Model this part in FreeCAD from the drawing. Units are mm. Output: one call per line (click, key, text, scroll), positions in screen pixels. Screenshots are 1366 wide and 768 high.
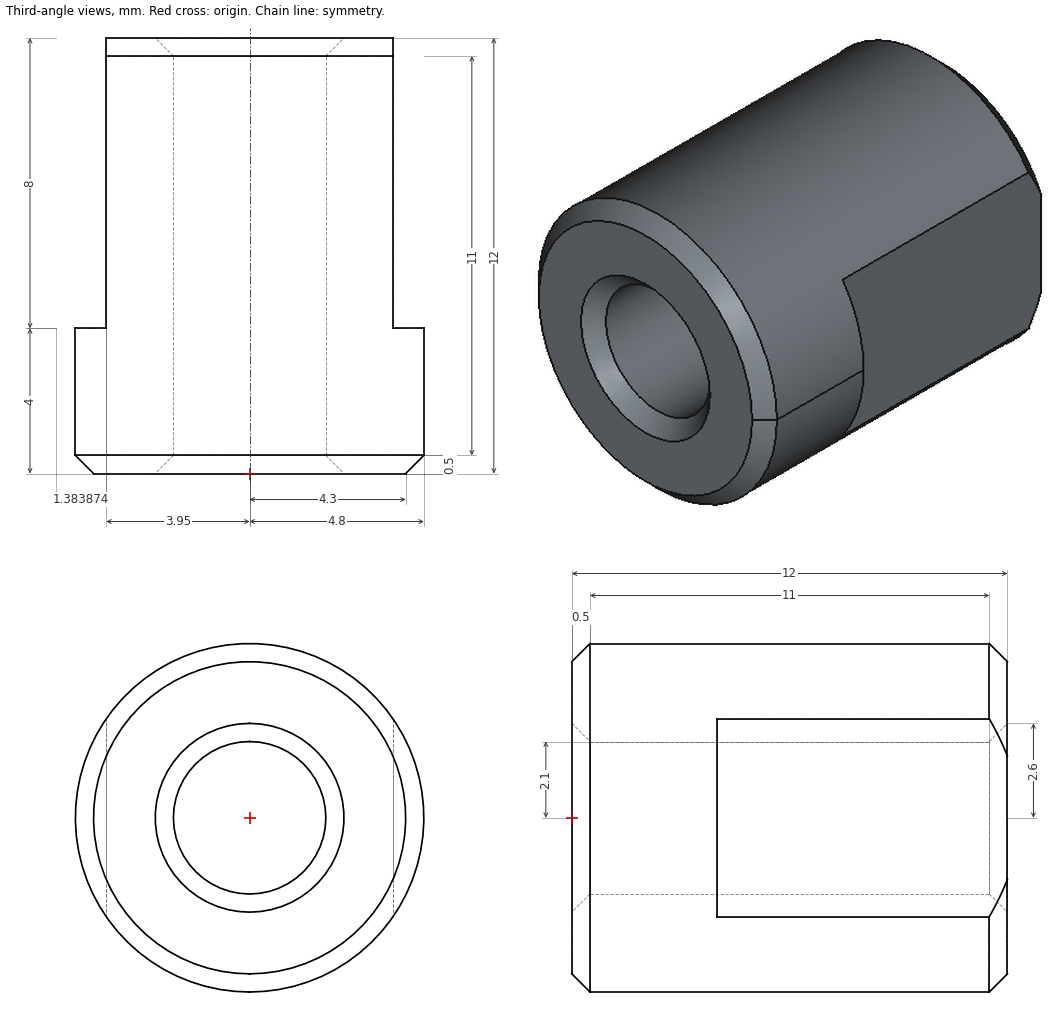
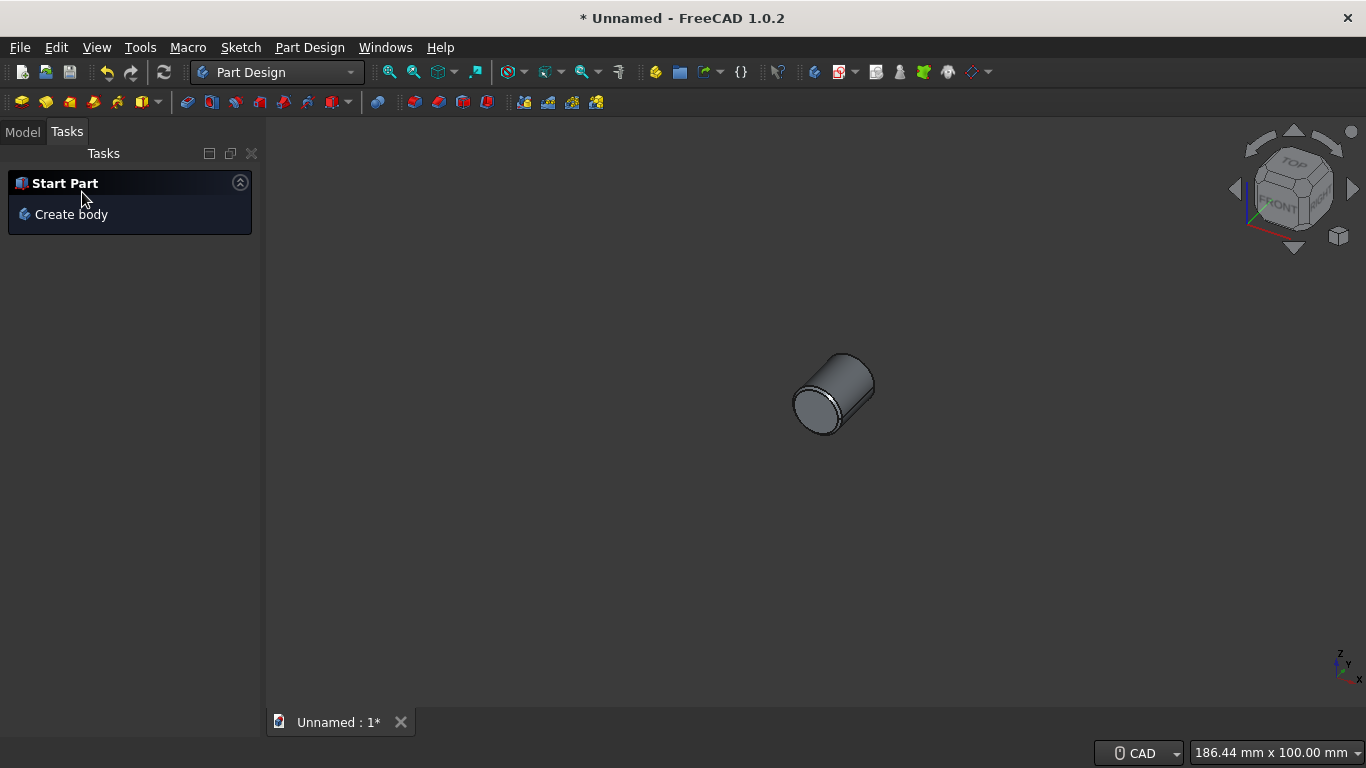
click(390, 72)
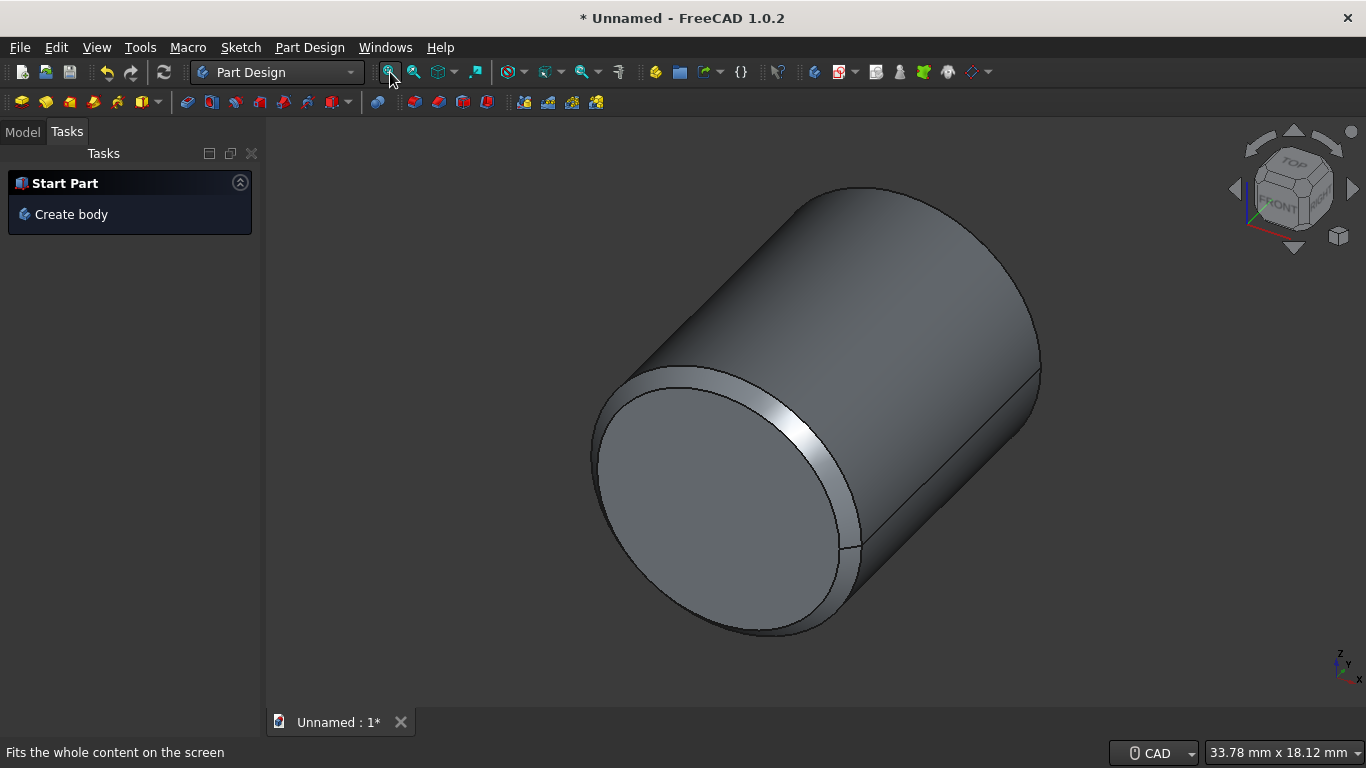
click(840, 72)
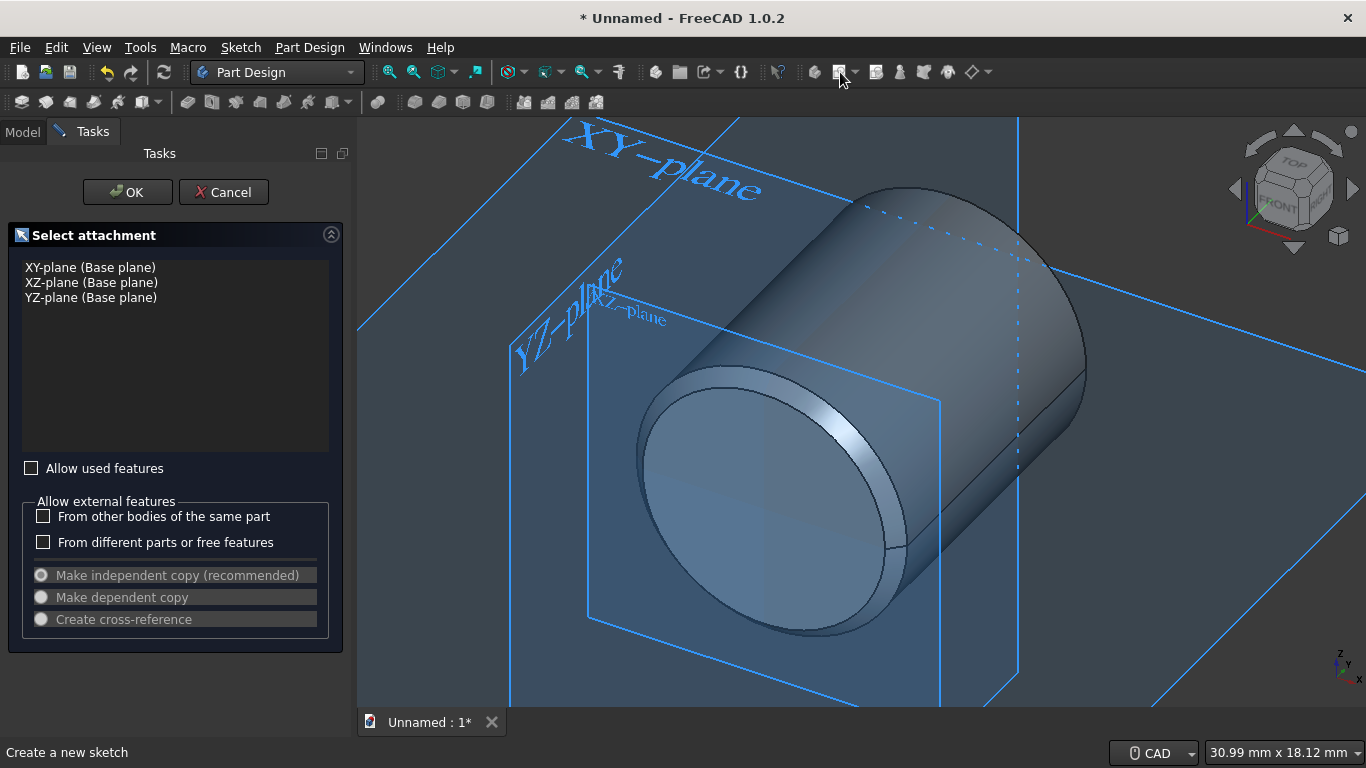
click(82, 298)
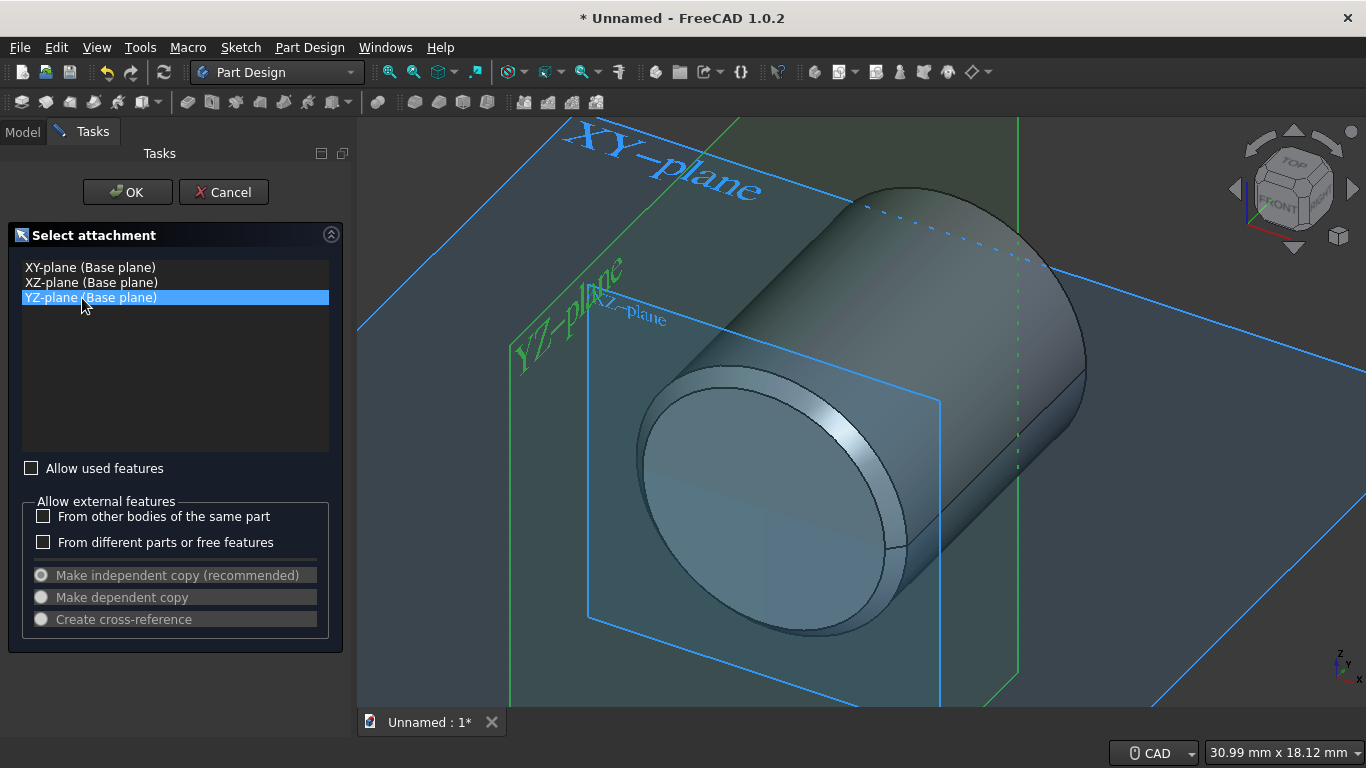
click(128, 192)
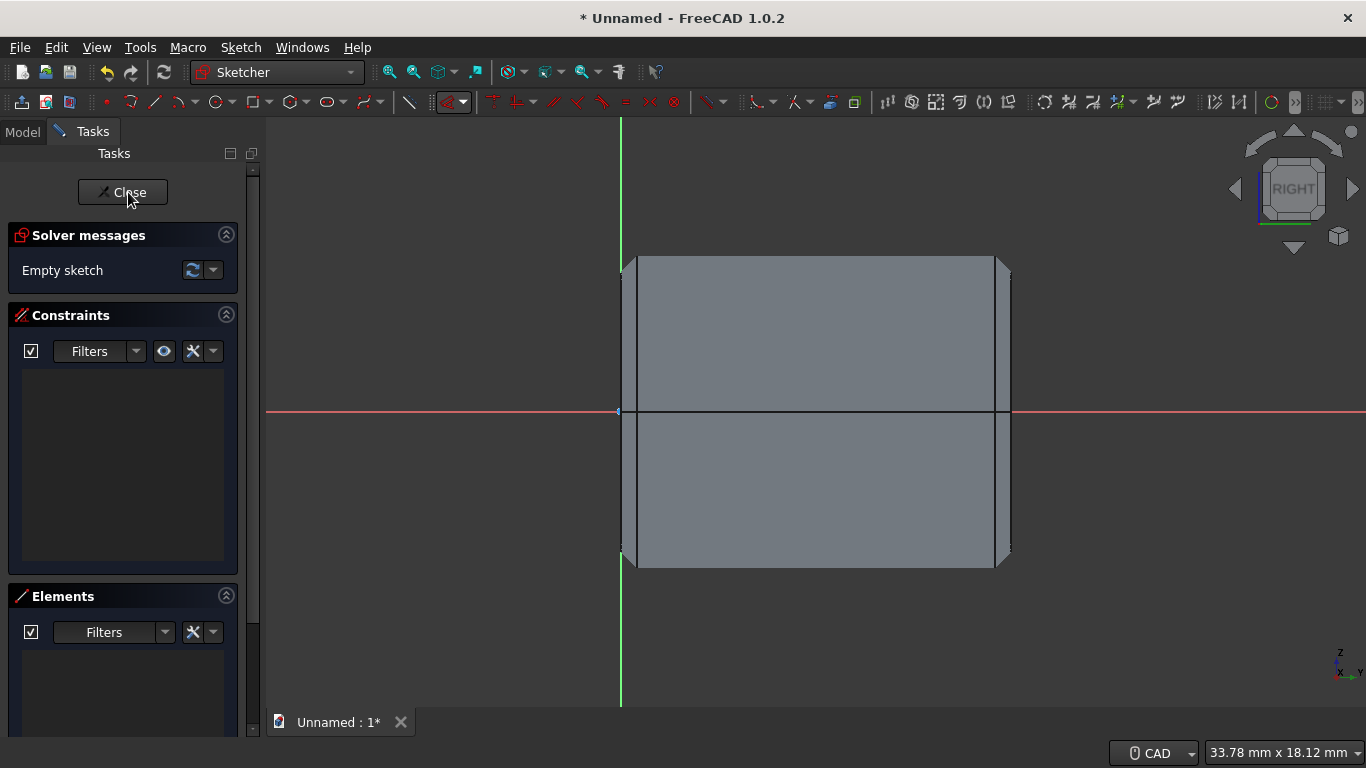
click(70, 102)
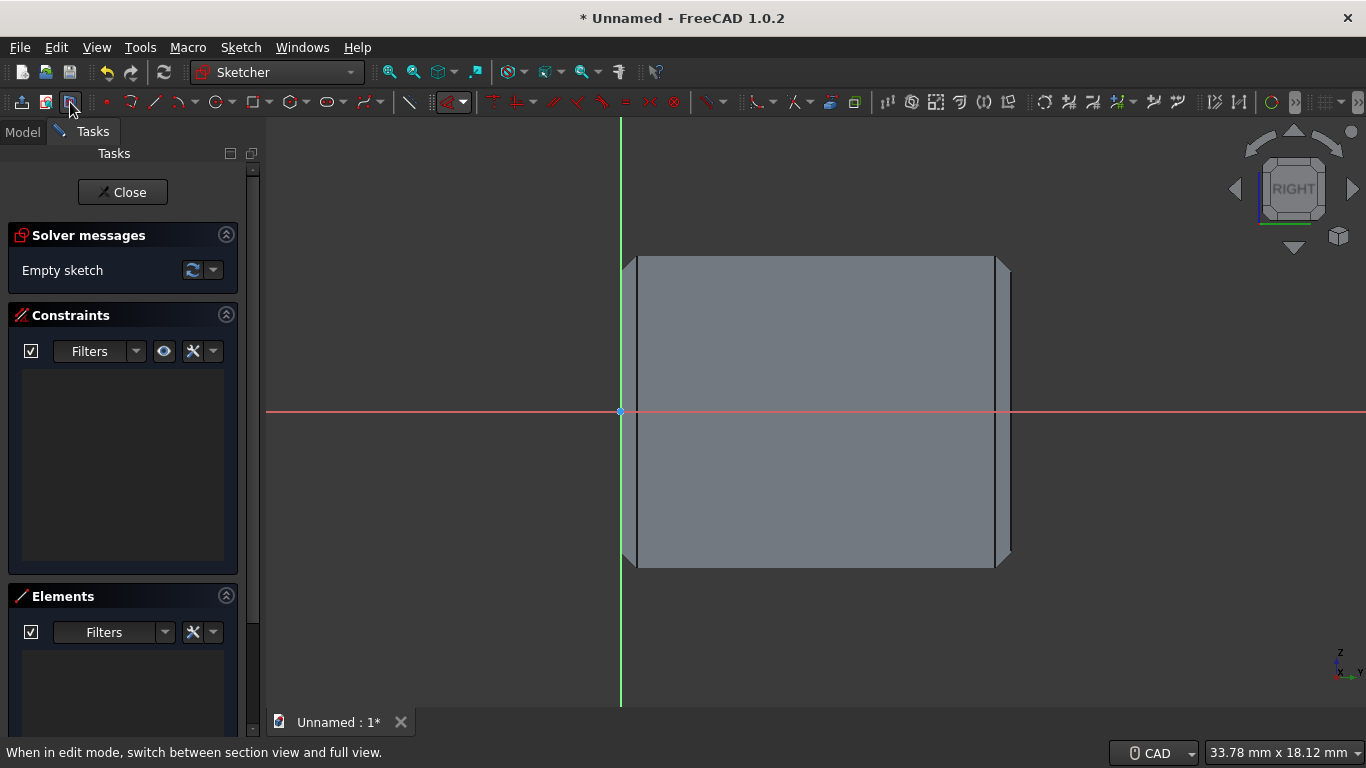
scroll(955, 284, up, 2)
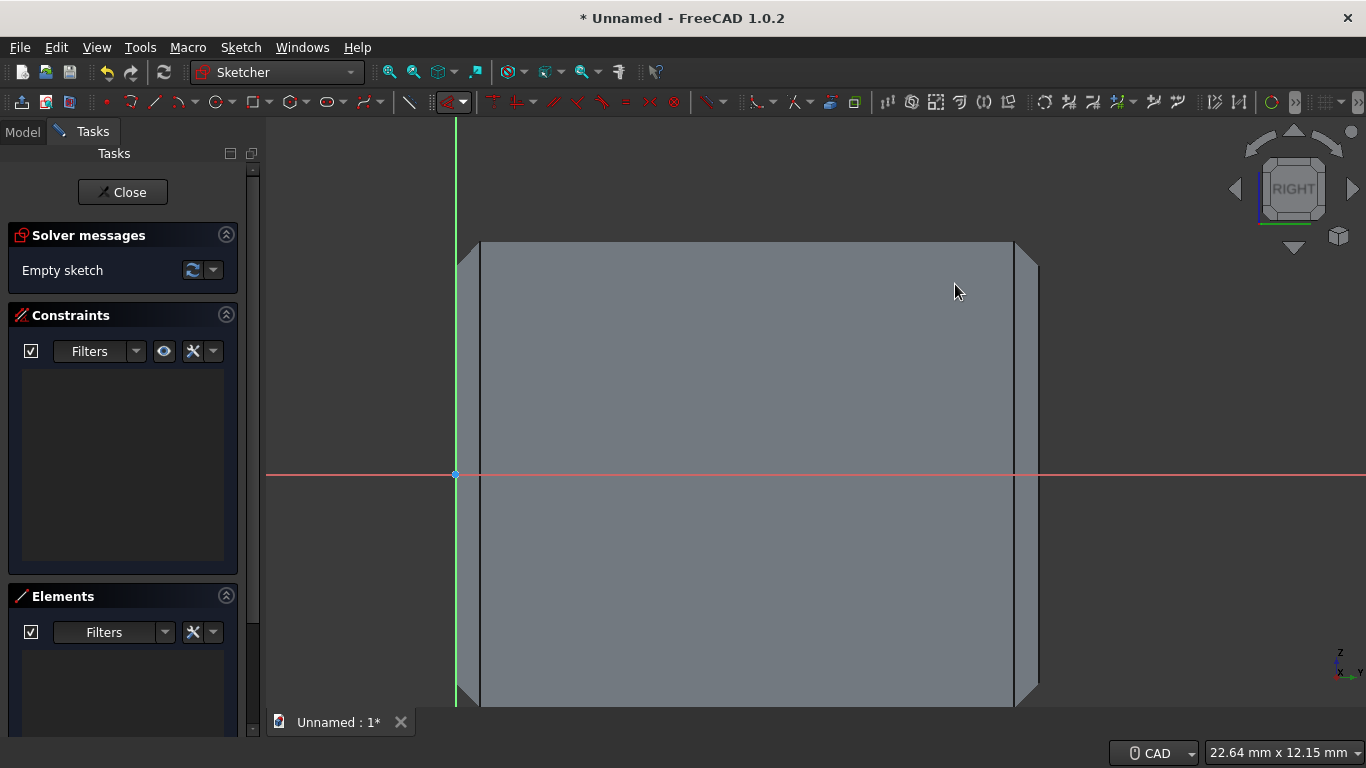
click(132, 102)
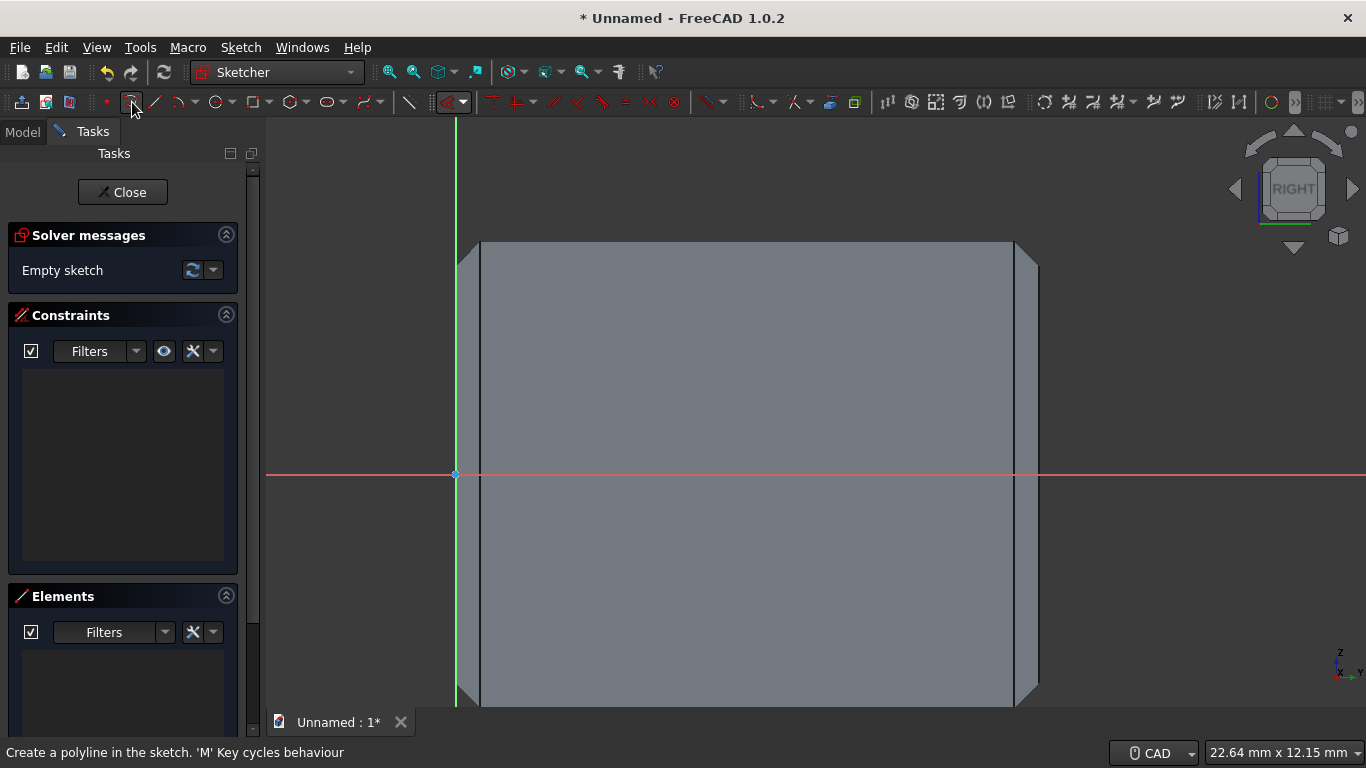
click(456, 475)
click(1039, 466)
click(1039, 349)
click(1014, 373)
click(480, 373)
click(465, 349)
click(456, 475)
key(Escape)
key(Escape)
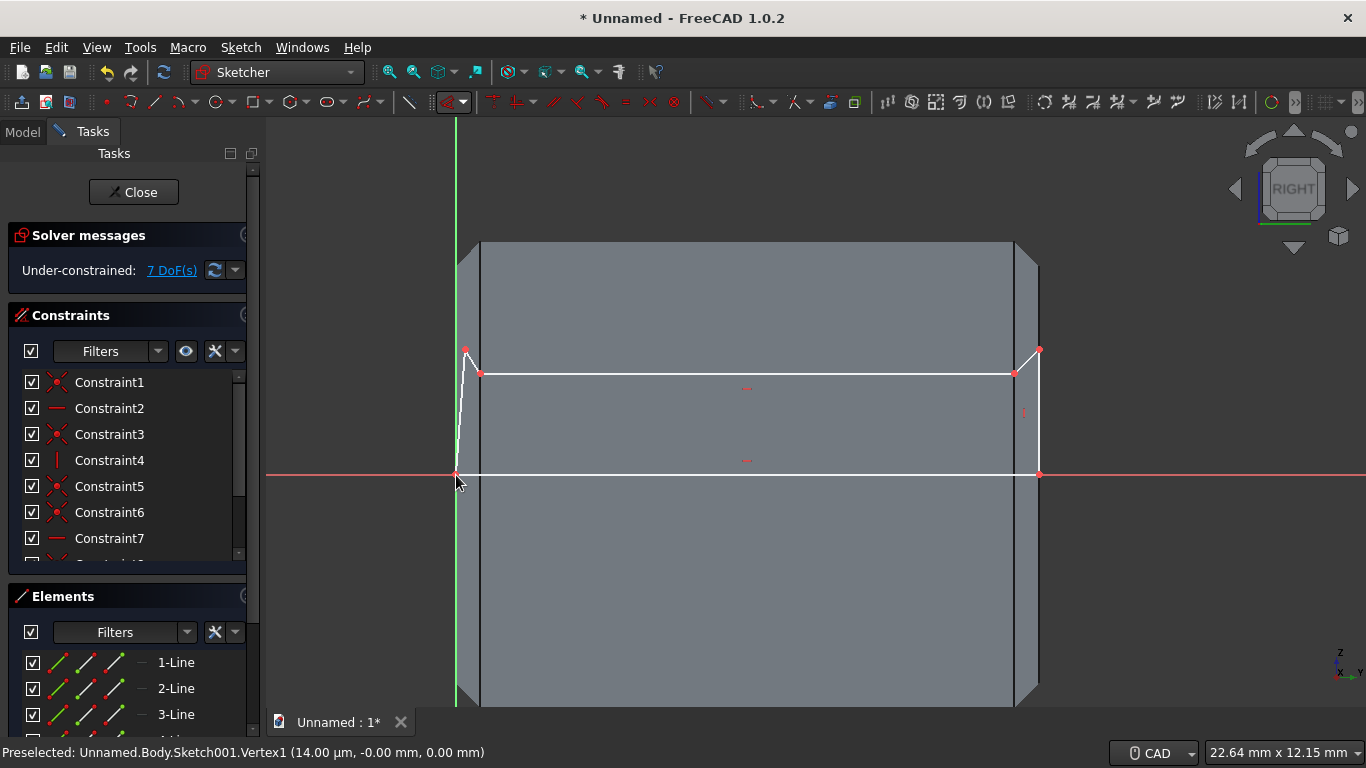
click(459, 437)